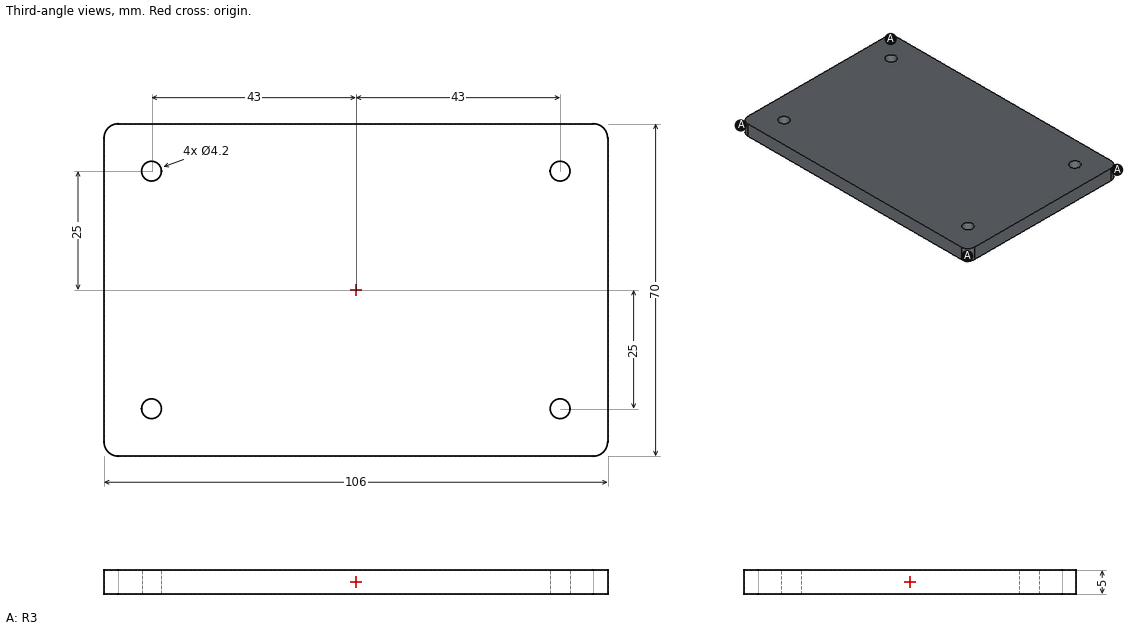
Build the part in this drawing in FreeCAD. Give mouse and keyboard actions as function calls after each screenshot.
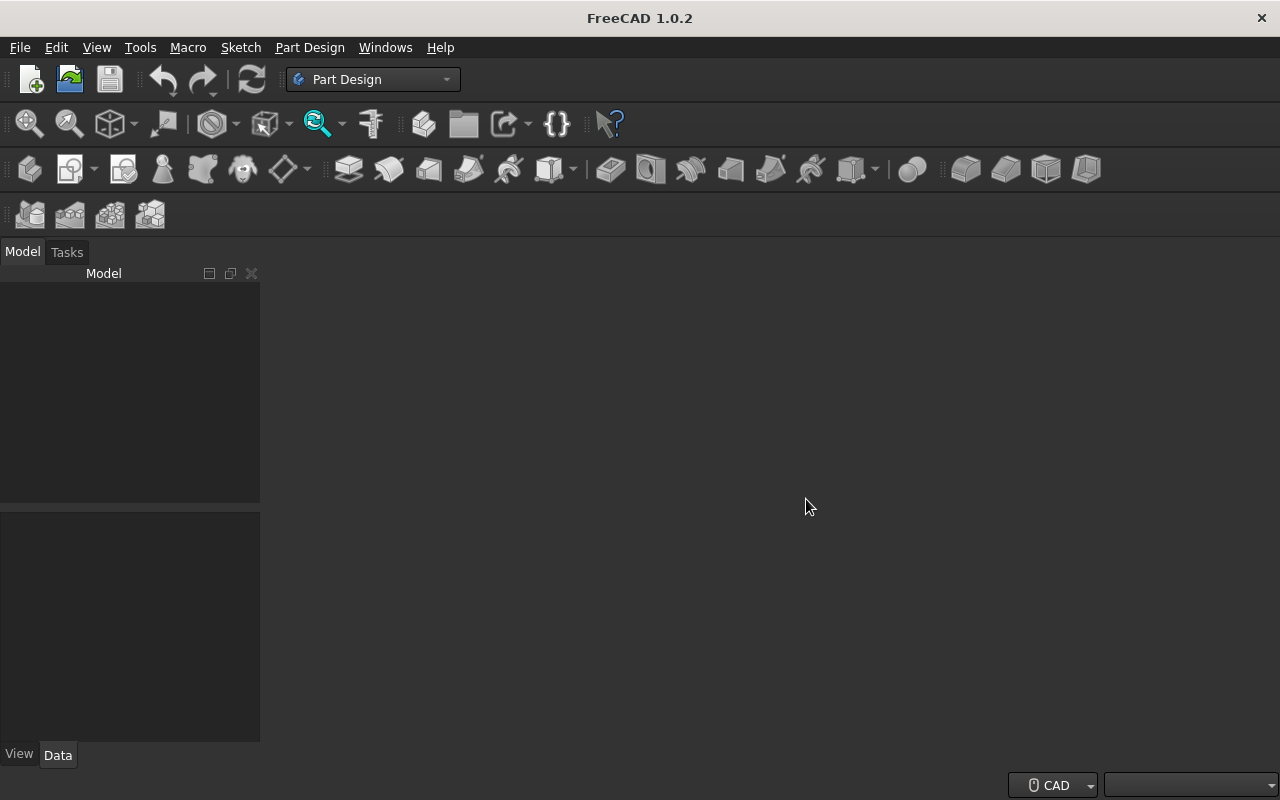
click(30, 80)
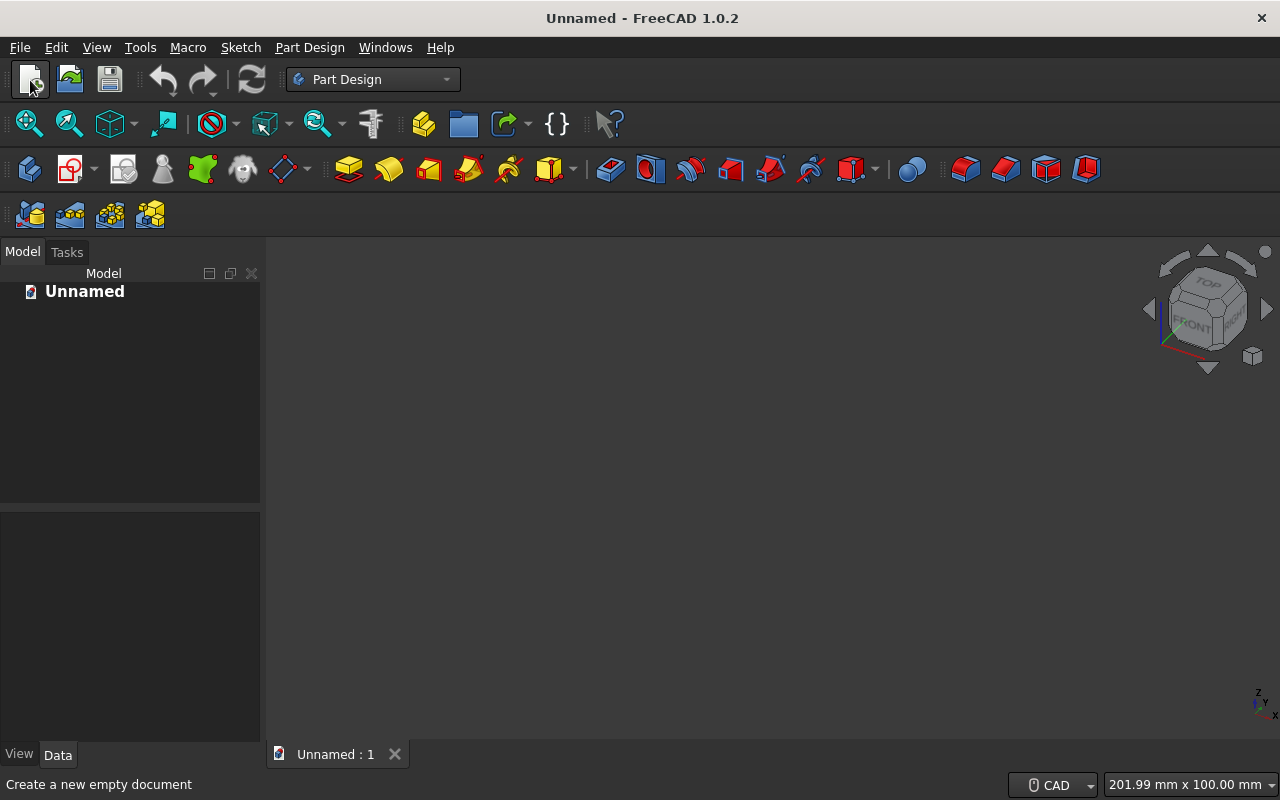
click(70, 170)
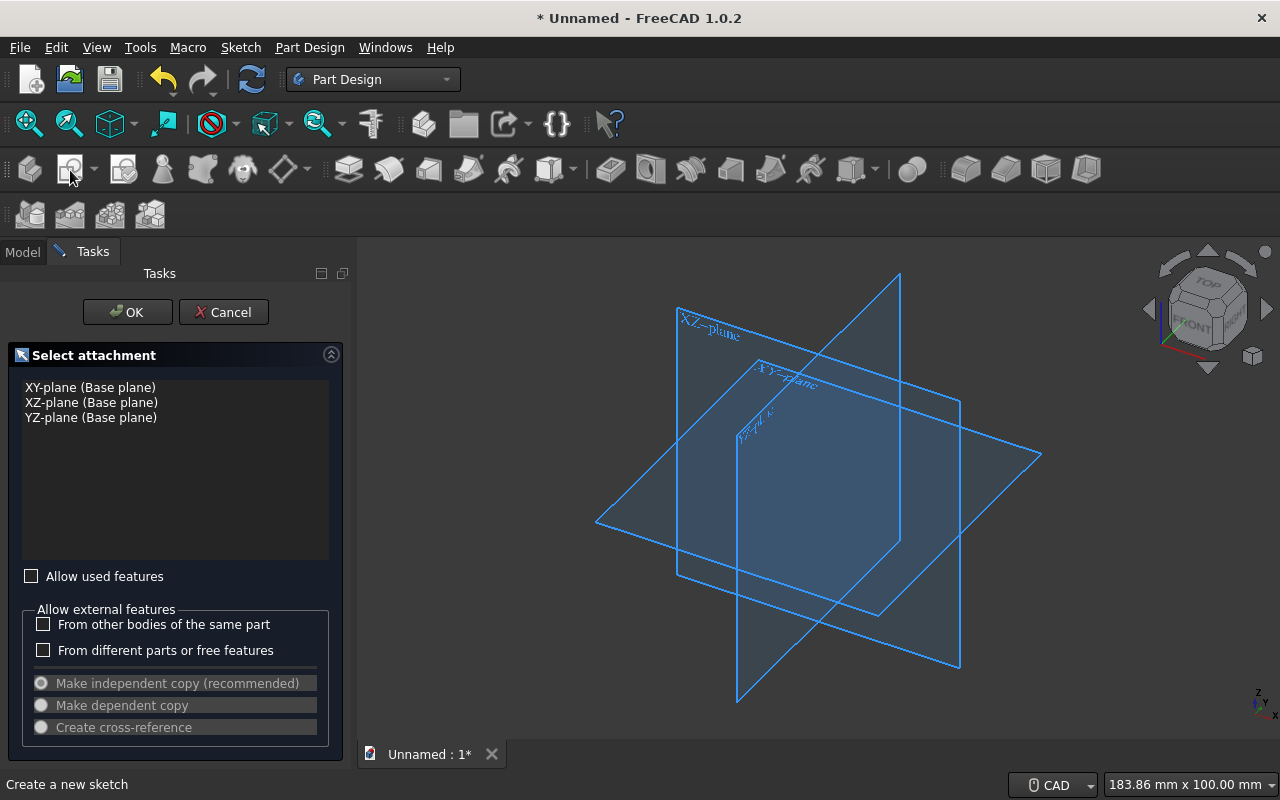
click(82, 388)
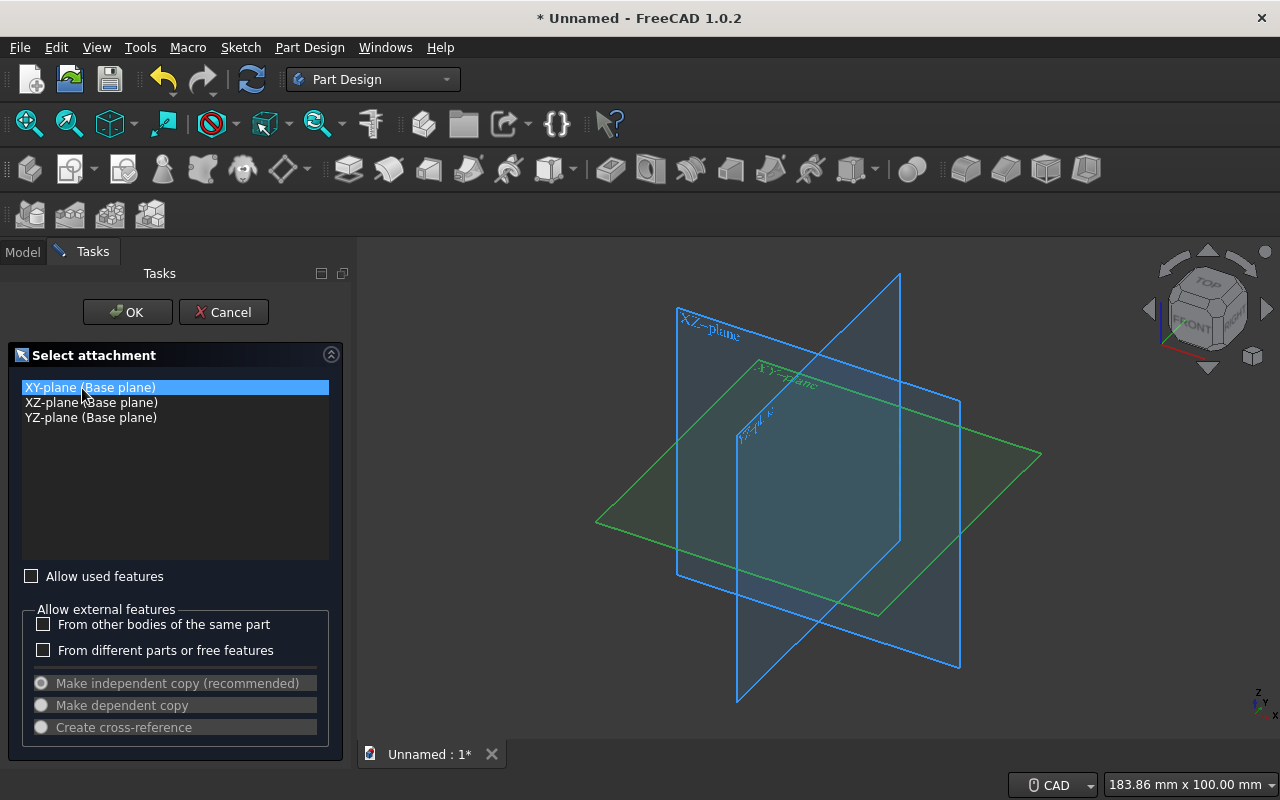
click(128, 312)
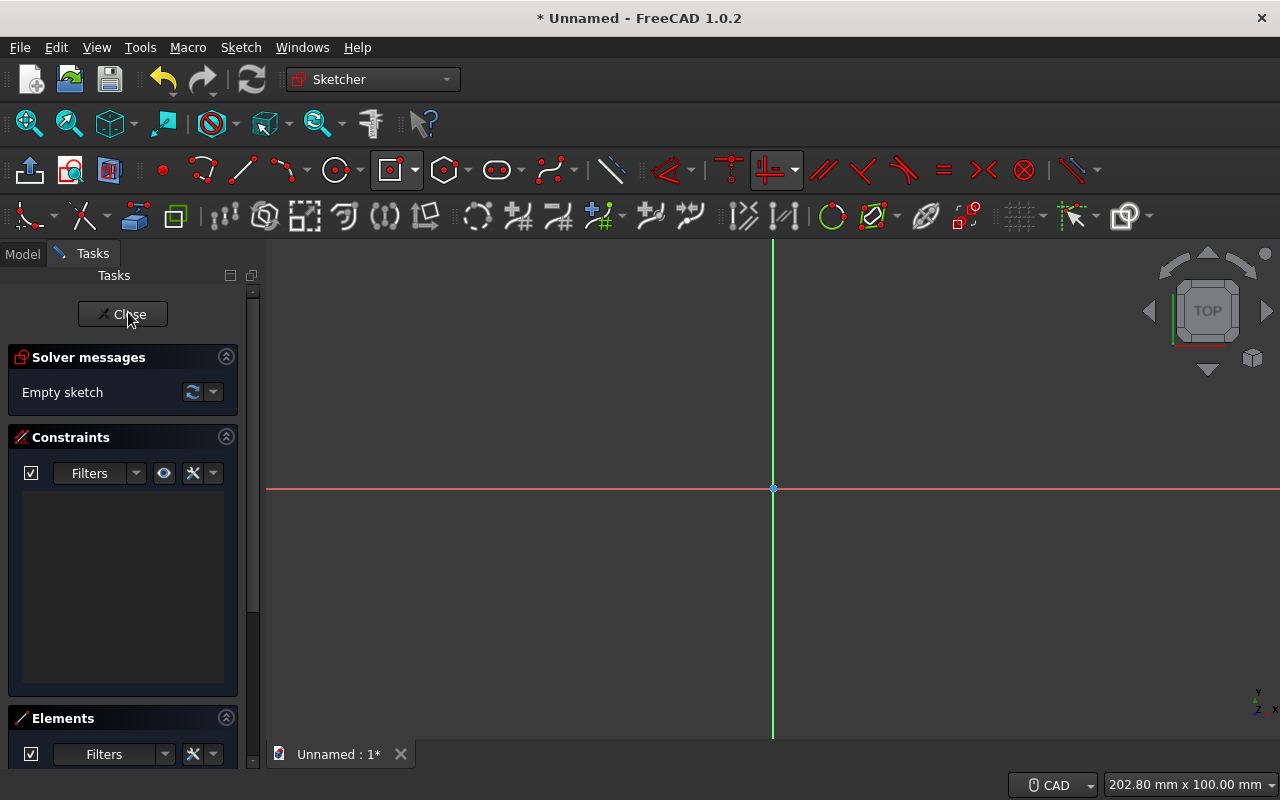
key(g)
key(v)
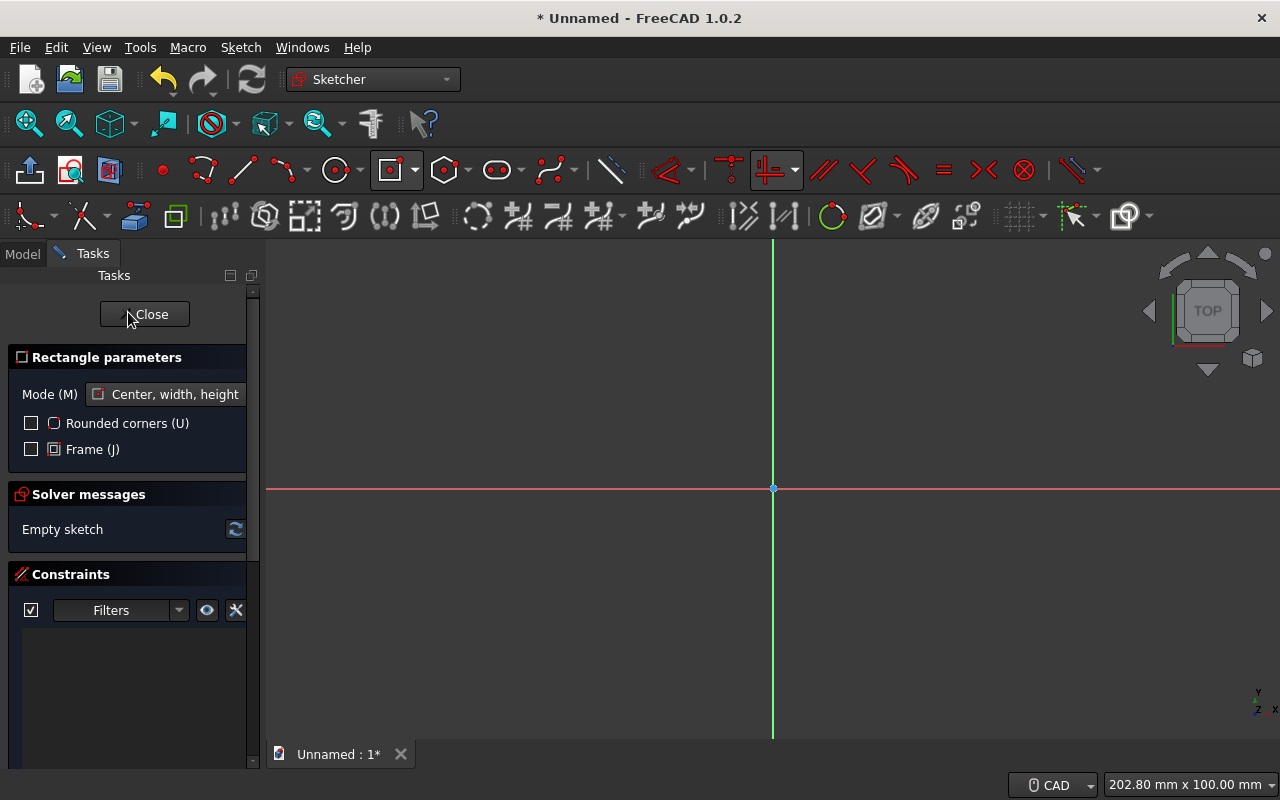
click(773, 489)
move(1038, 314)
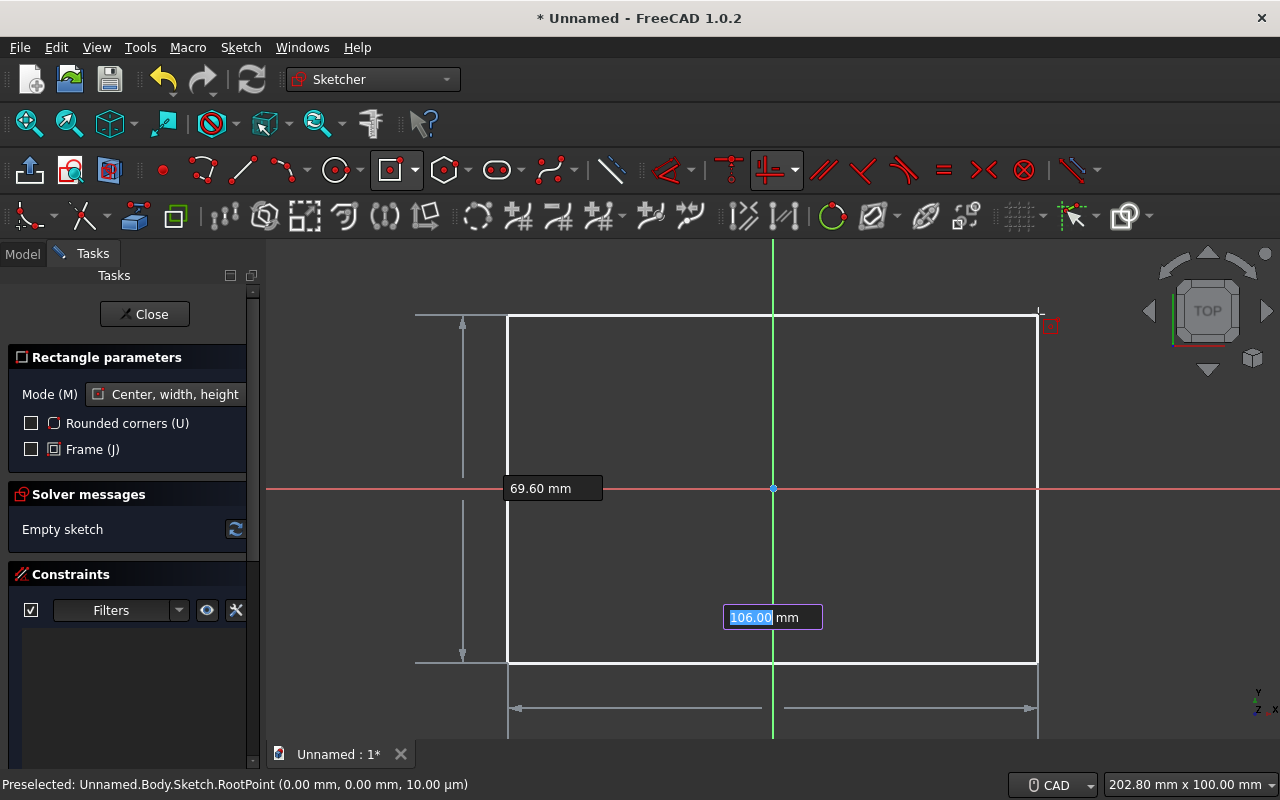
text(106)
key(Tab)
text(70)
key(Return)
key(Escape)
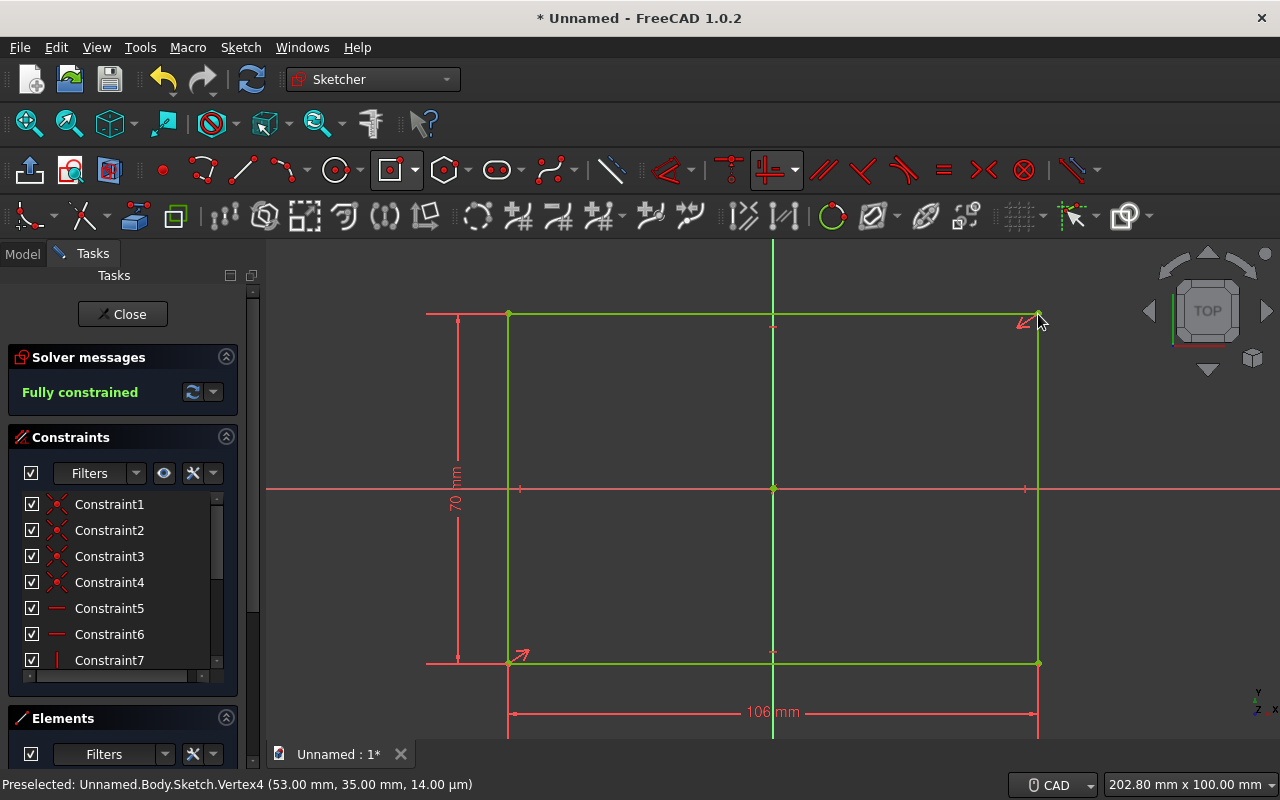
click(123, 314)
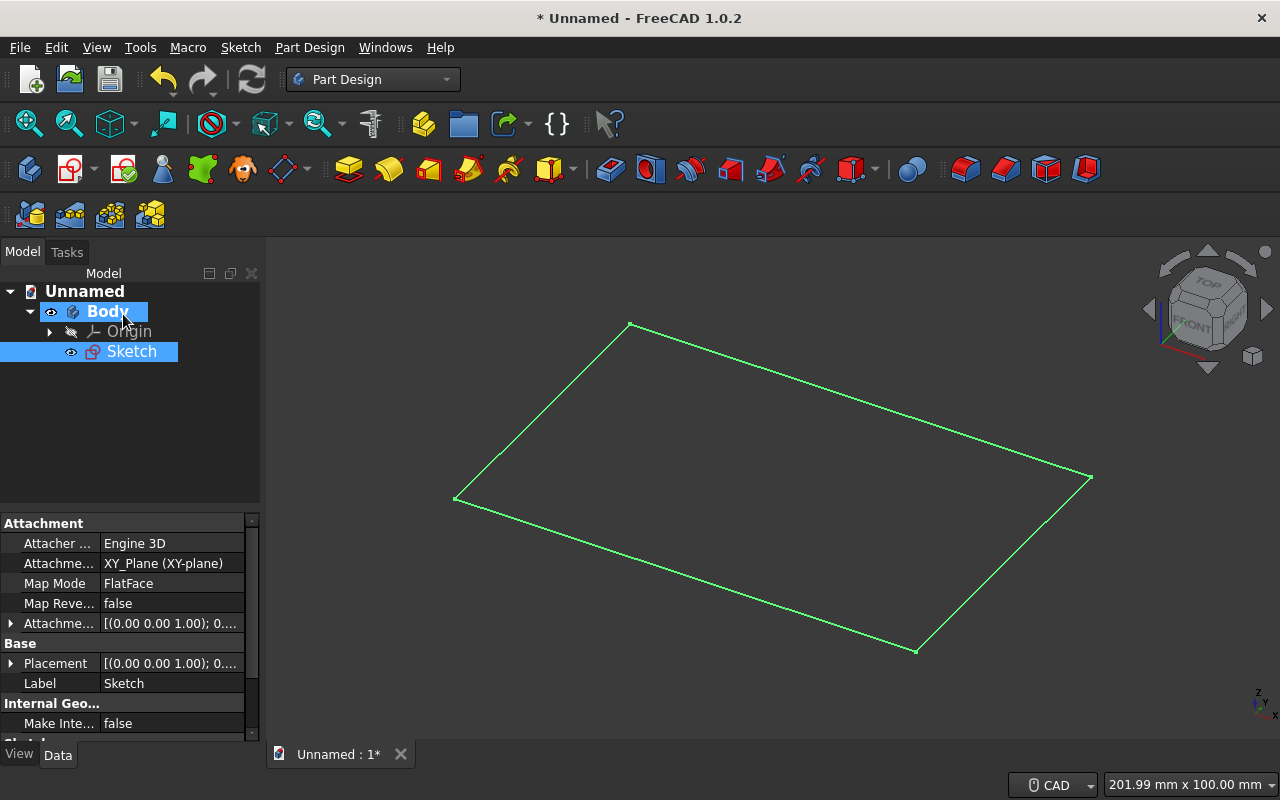
click(350, 170)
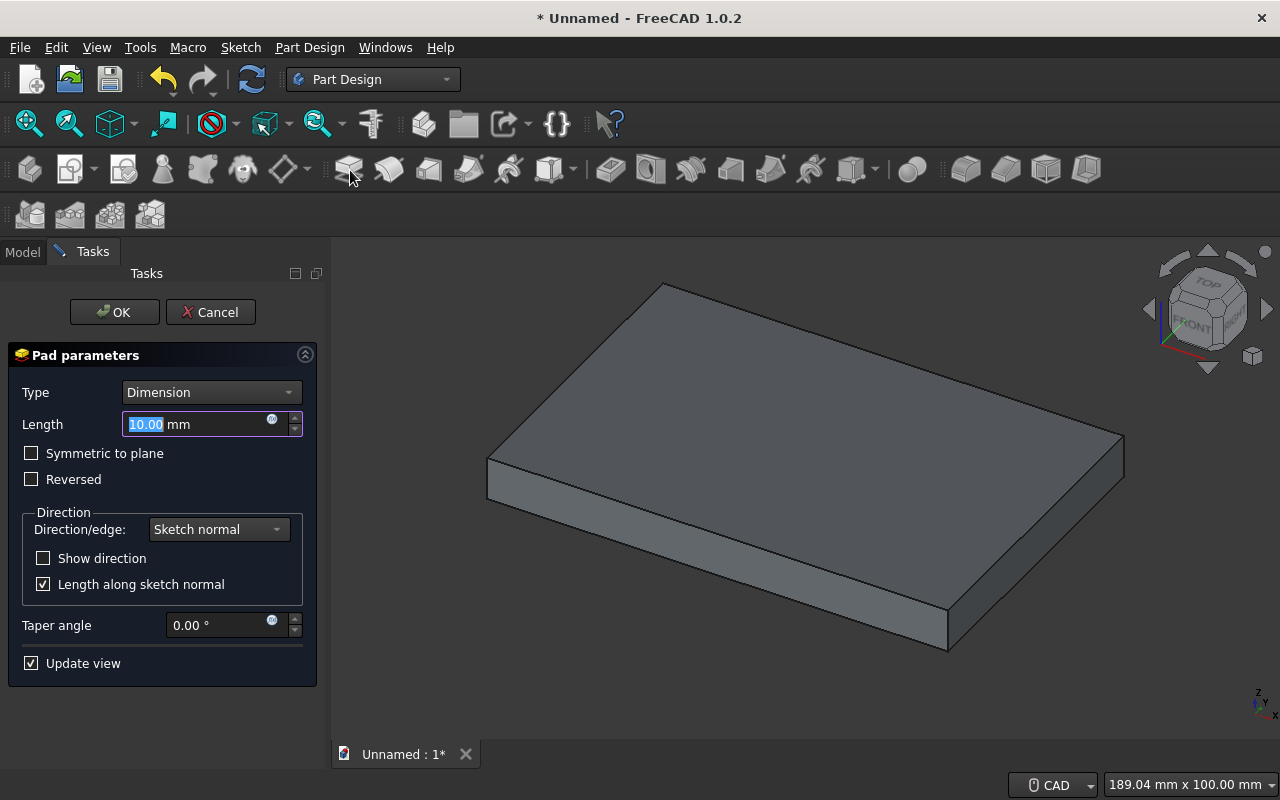
text(5)
key(Tab)